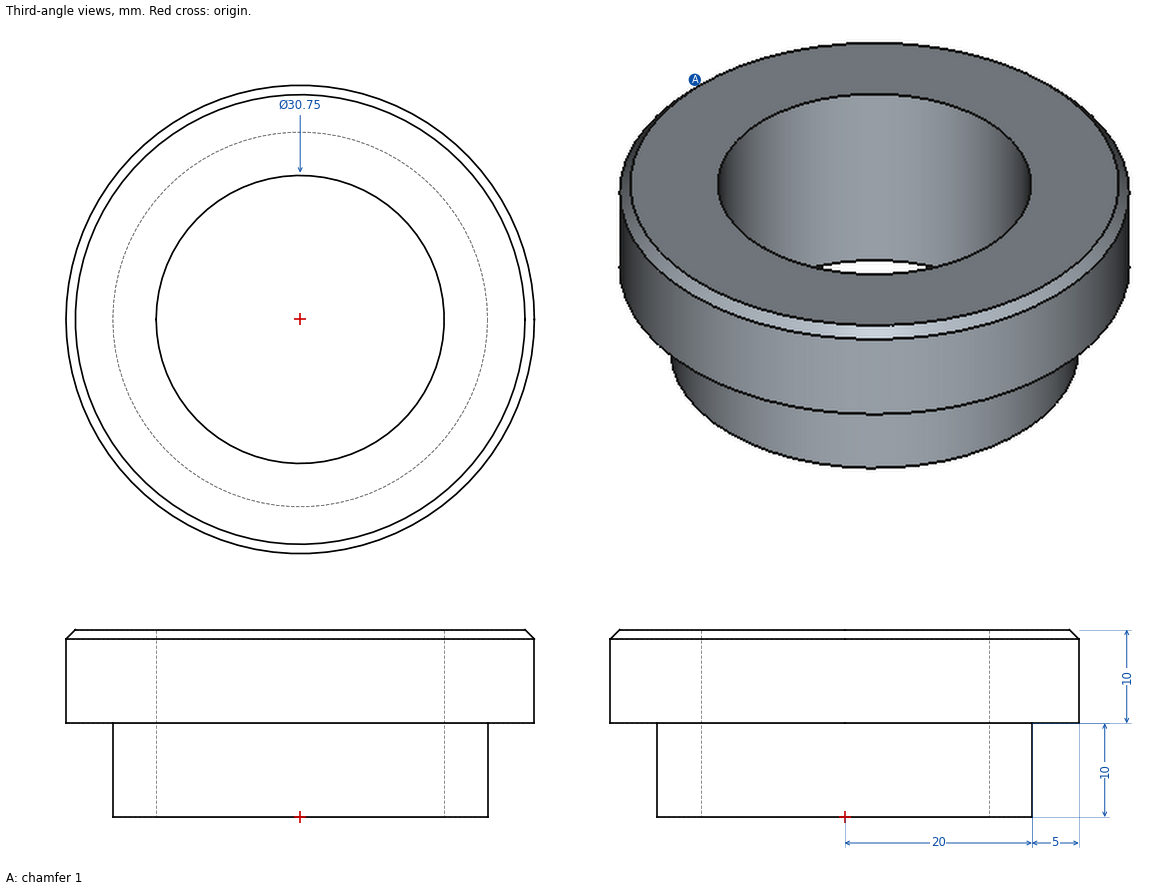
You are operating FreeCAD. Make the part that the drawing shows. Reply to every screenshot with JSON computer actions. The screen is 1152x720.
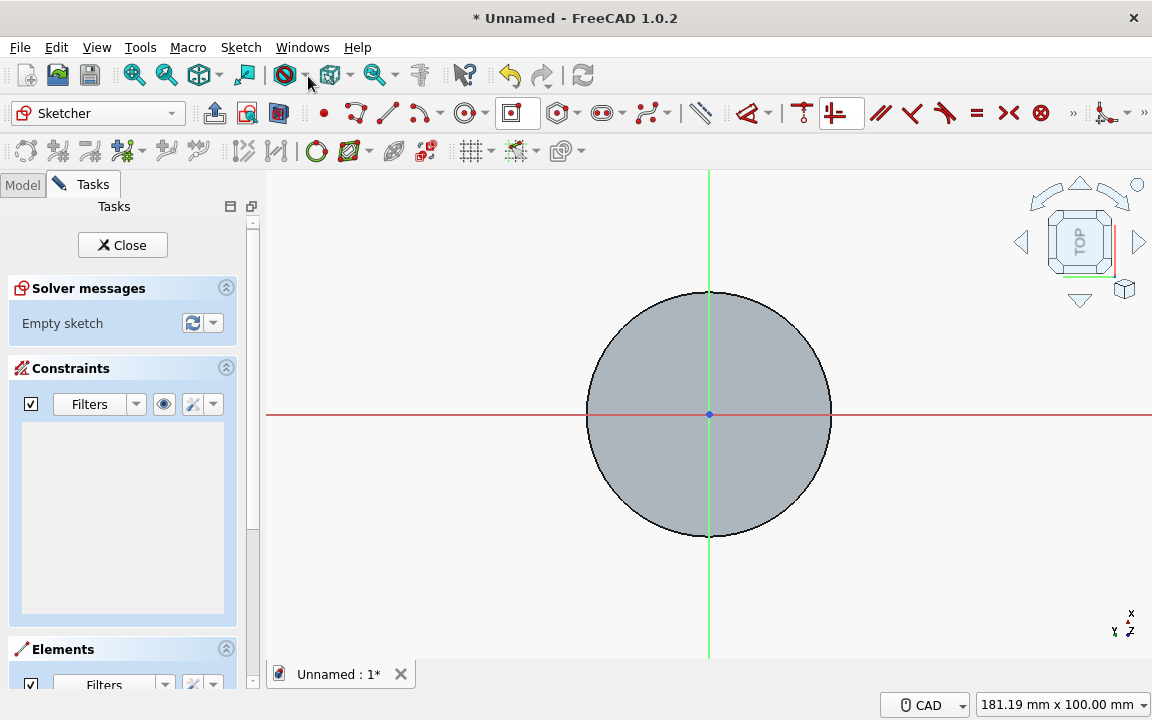
{"action": "scroll", "coordinate": [765, 415], "scroll_direction": "up", "scroll_amount": 4}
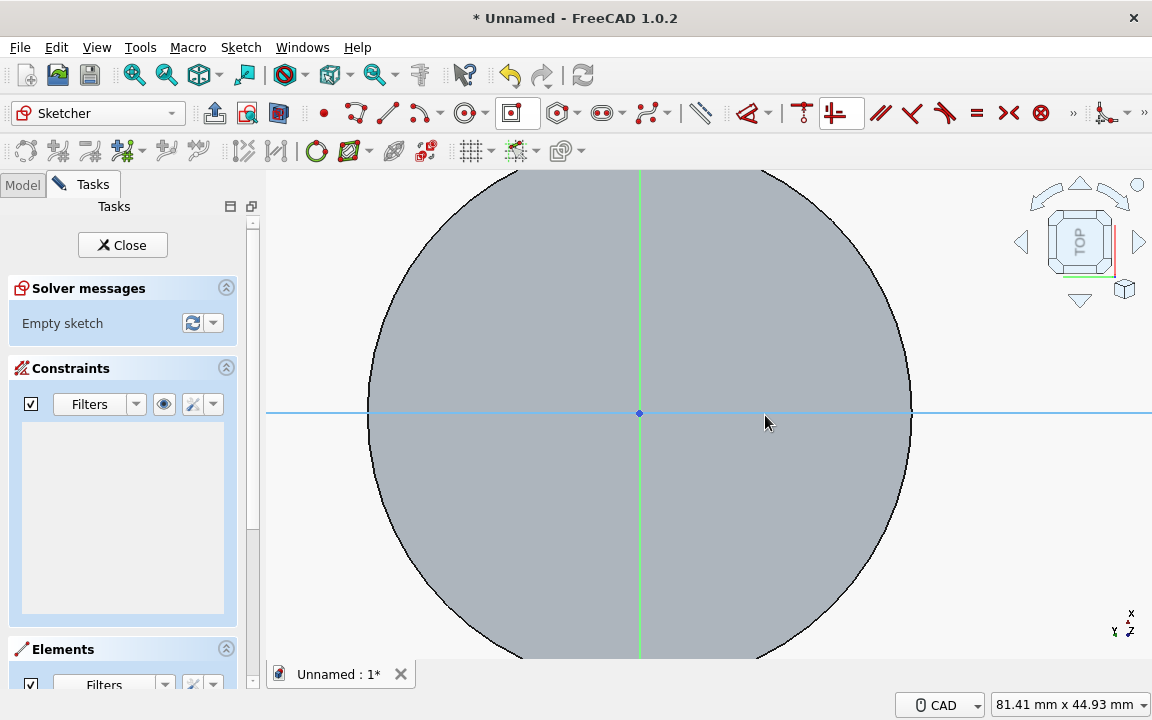
{"action": "key", "text": "g c"}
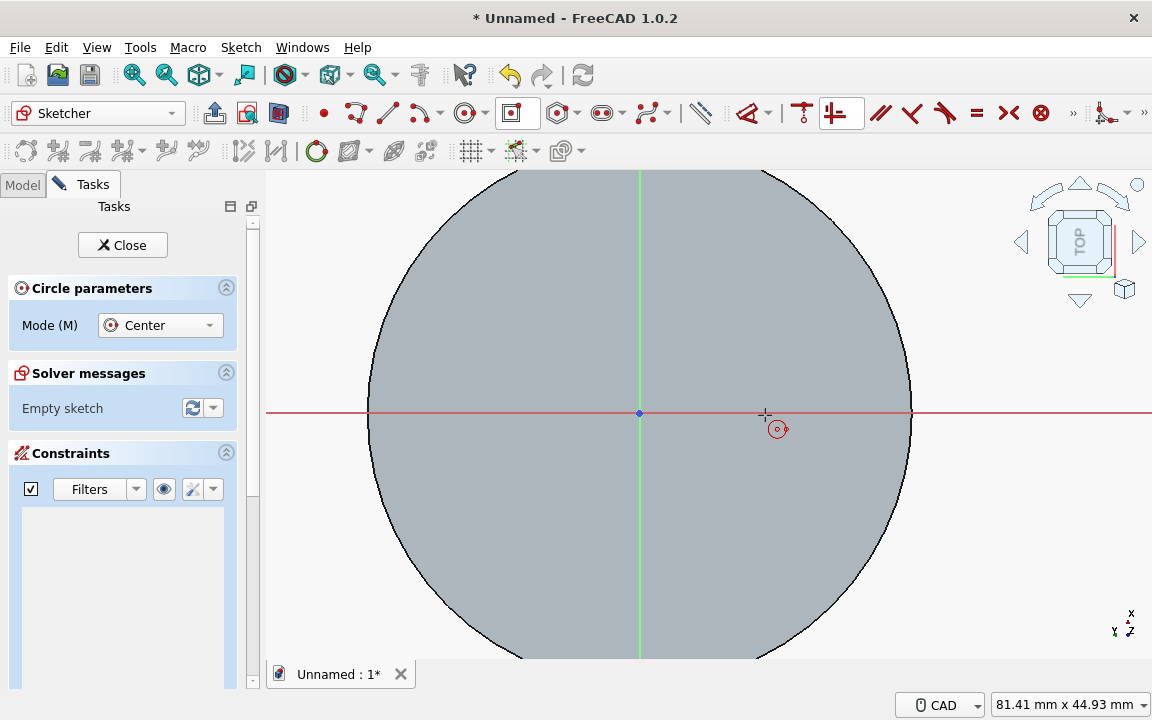
{"action": "left_click", "coordinate": [640, 413]}
{"action": "left_click", "coordinate": [758, 295]}
{"action": "key", "text": "Escape"}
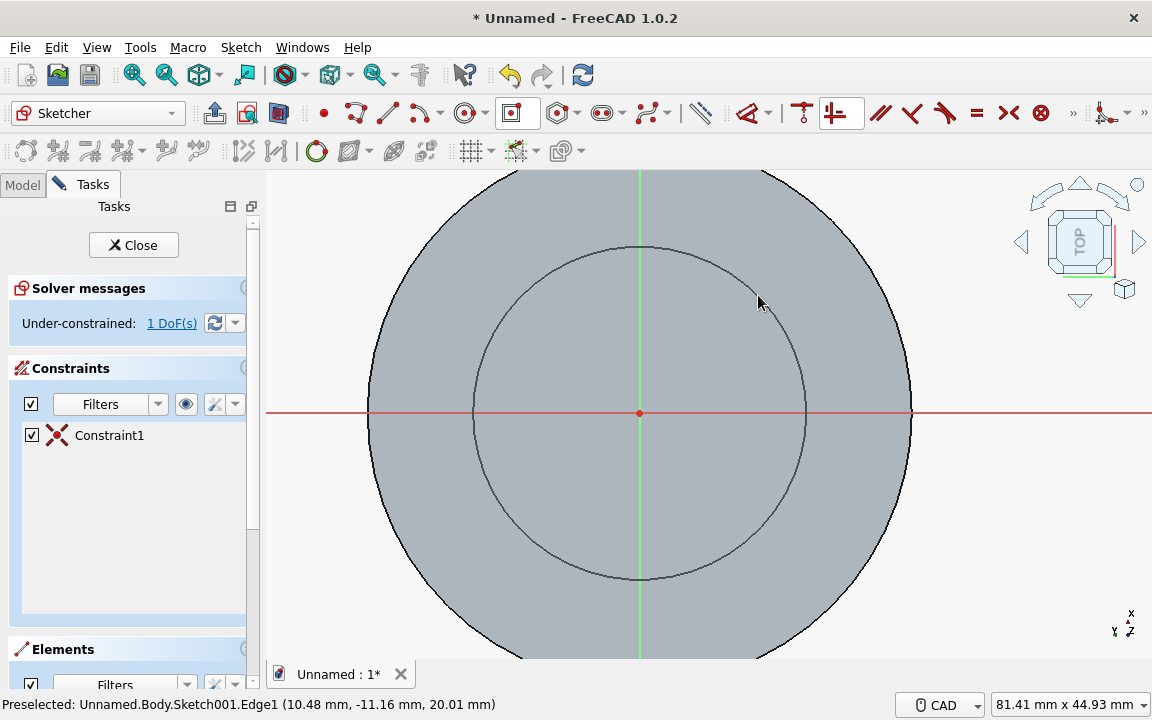
{"action": "left_click", "coordinate": [757, 295]}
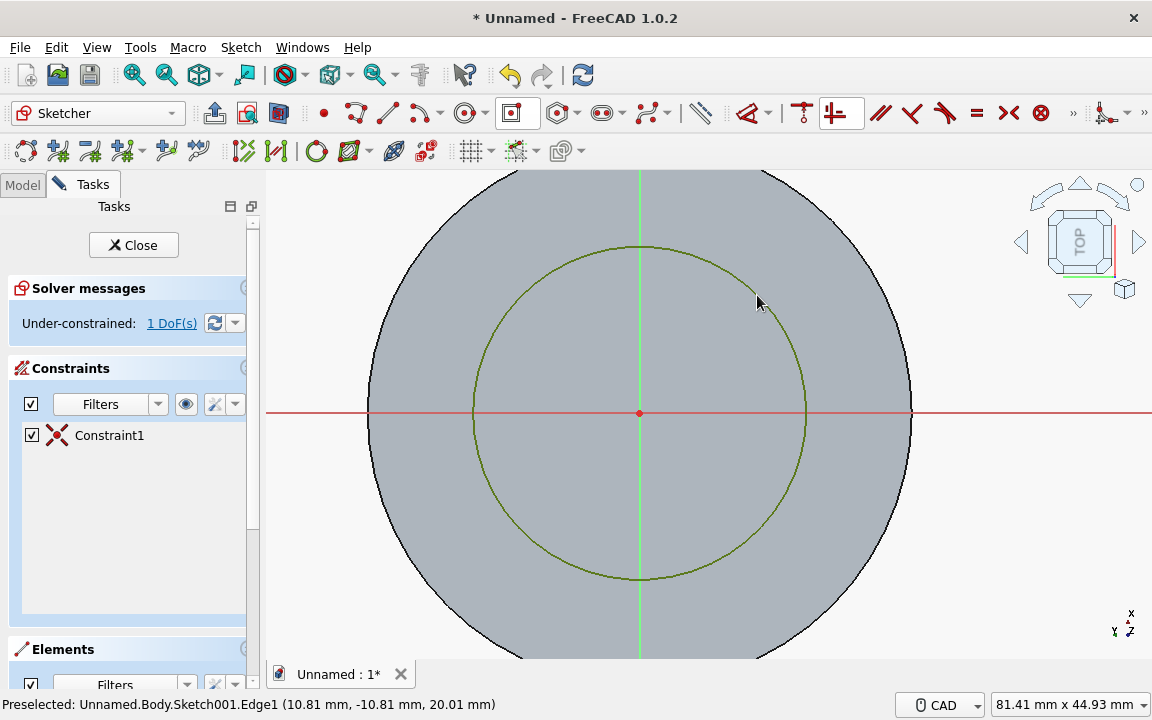
{"action": "key", "text": "k o"}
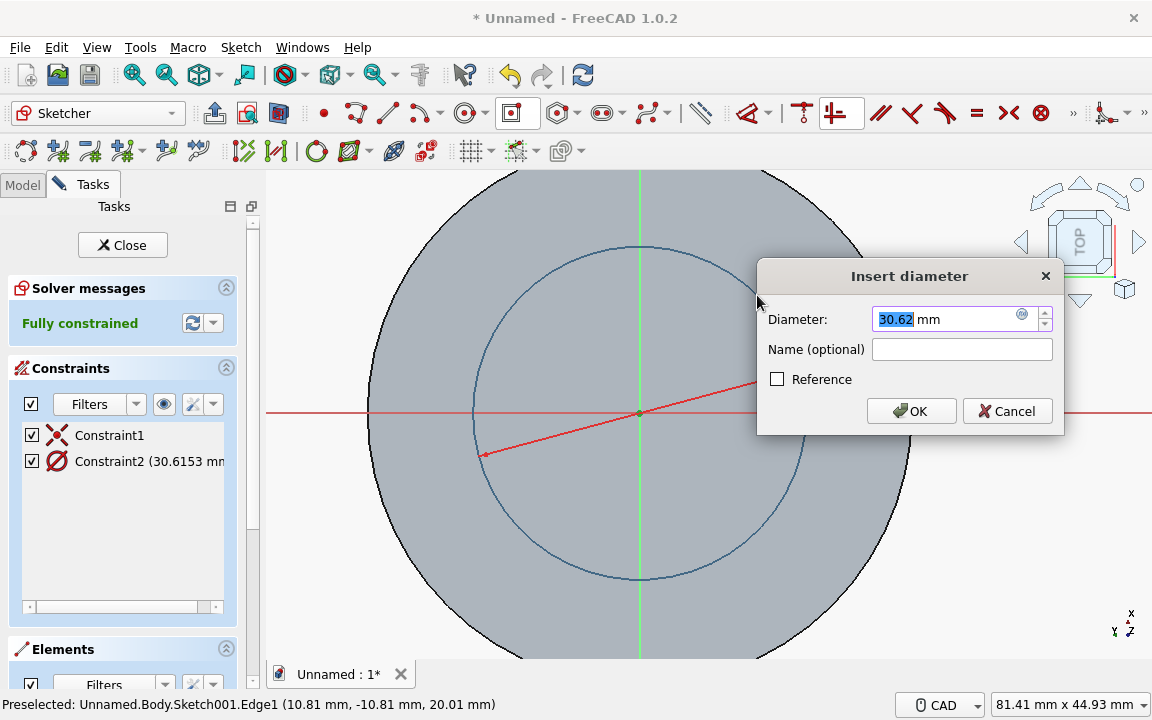
{"action": "type", "text": "30.75"}
{"action": "key", "text": "Return"}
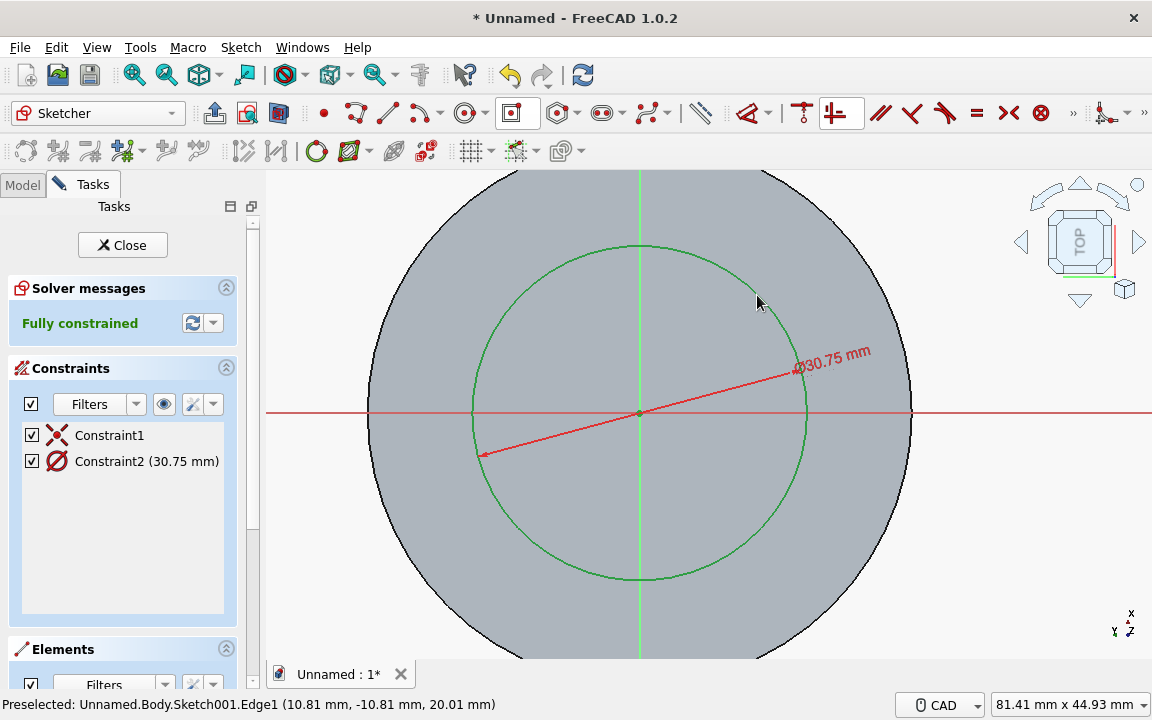
{"action": "left_click", "coordinate": [123, 245]}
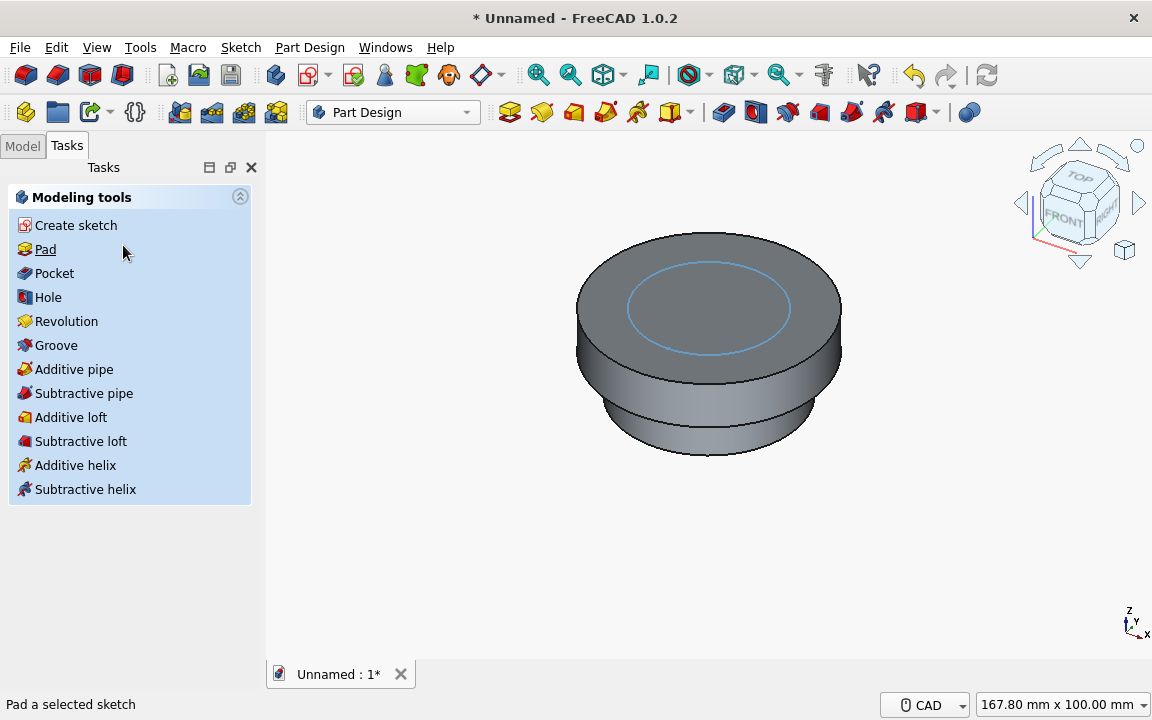
{"action": "left_click", "coordinate": [724, 112]}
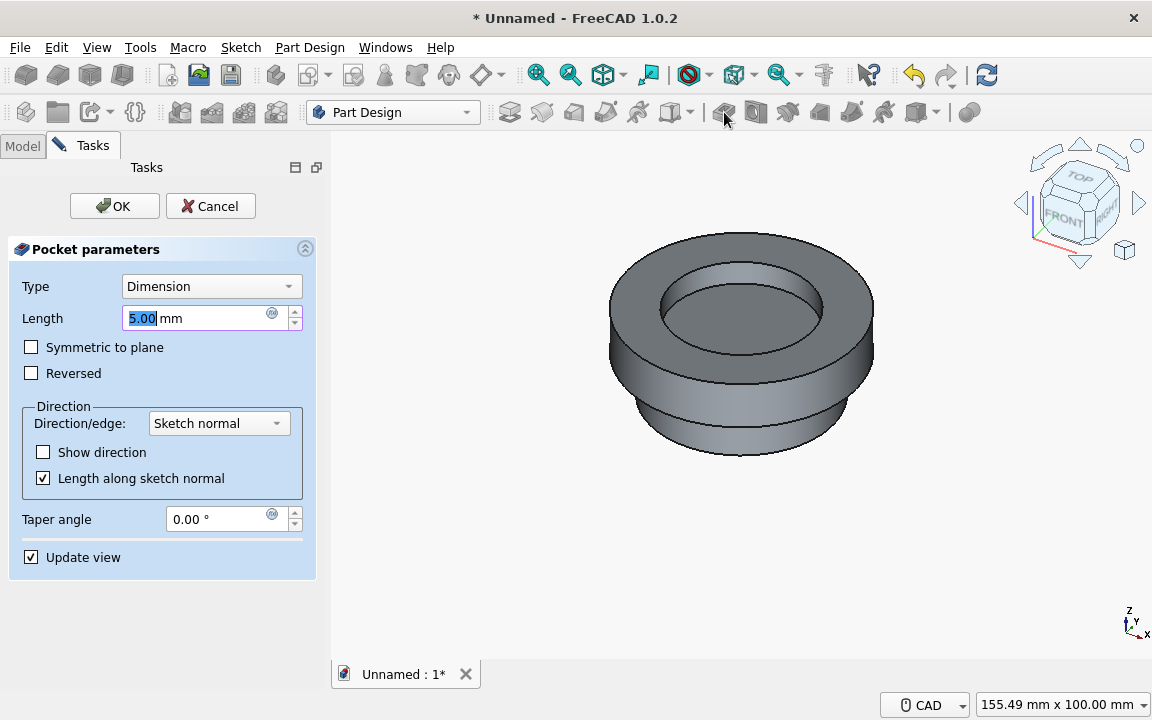
{"action": "left_click", "coordinate": [212, 286]}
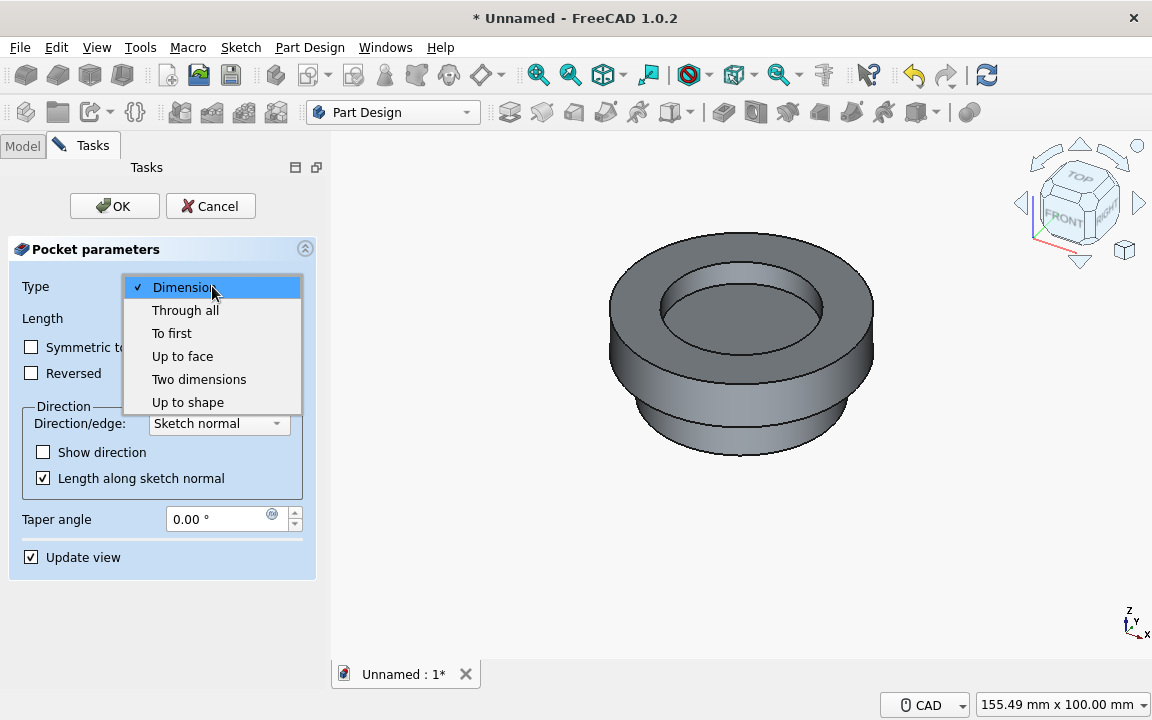
{"action": "left_click", "coordinate": [212, 310]}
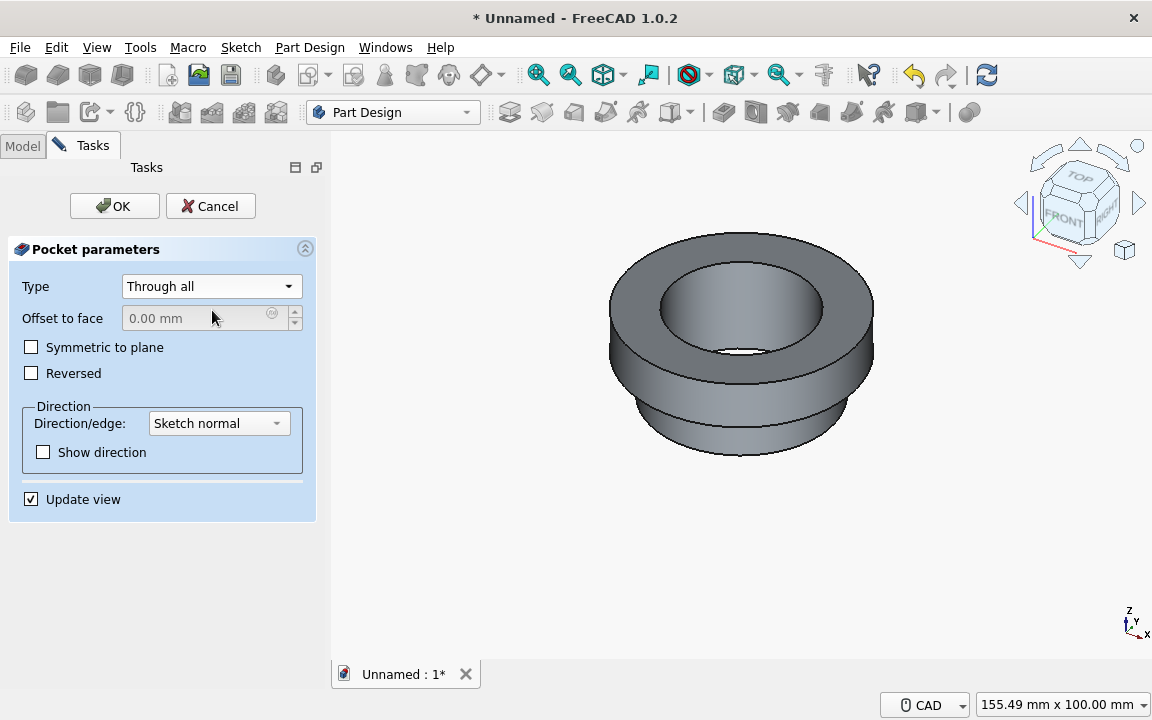
{"action": "left_click", "coordinate": [115, 206]}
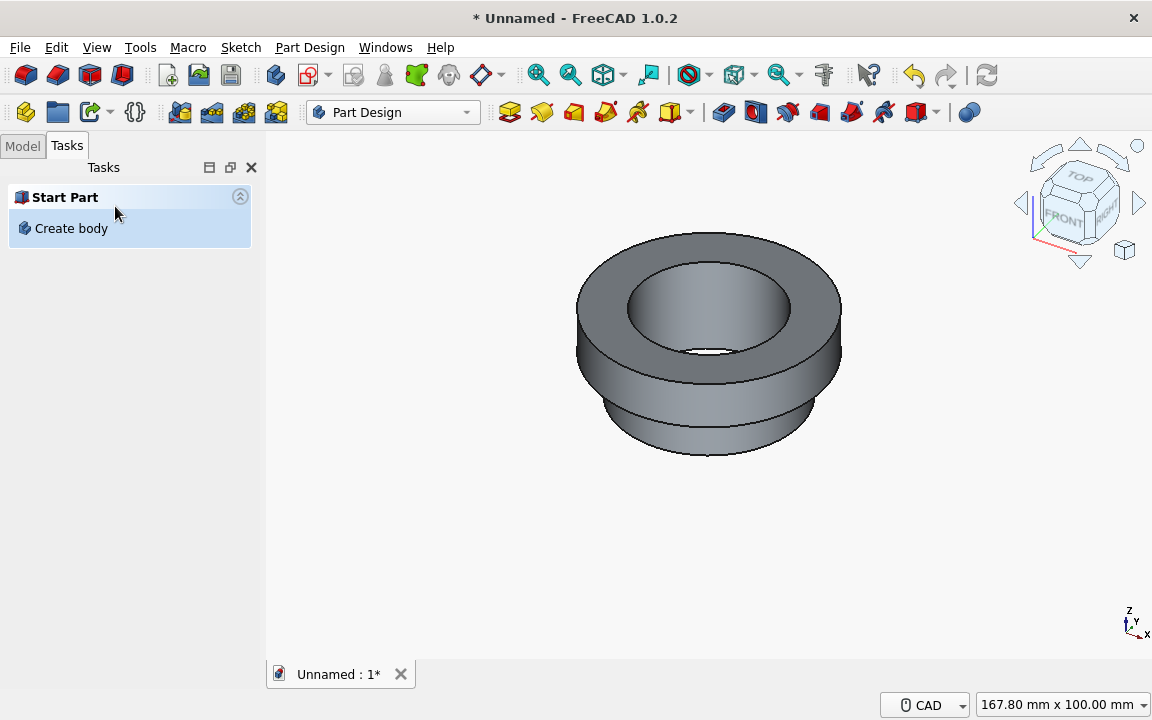
{"action": "left_click", "coordinate": [643, 373]}